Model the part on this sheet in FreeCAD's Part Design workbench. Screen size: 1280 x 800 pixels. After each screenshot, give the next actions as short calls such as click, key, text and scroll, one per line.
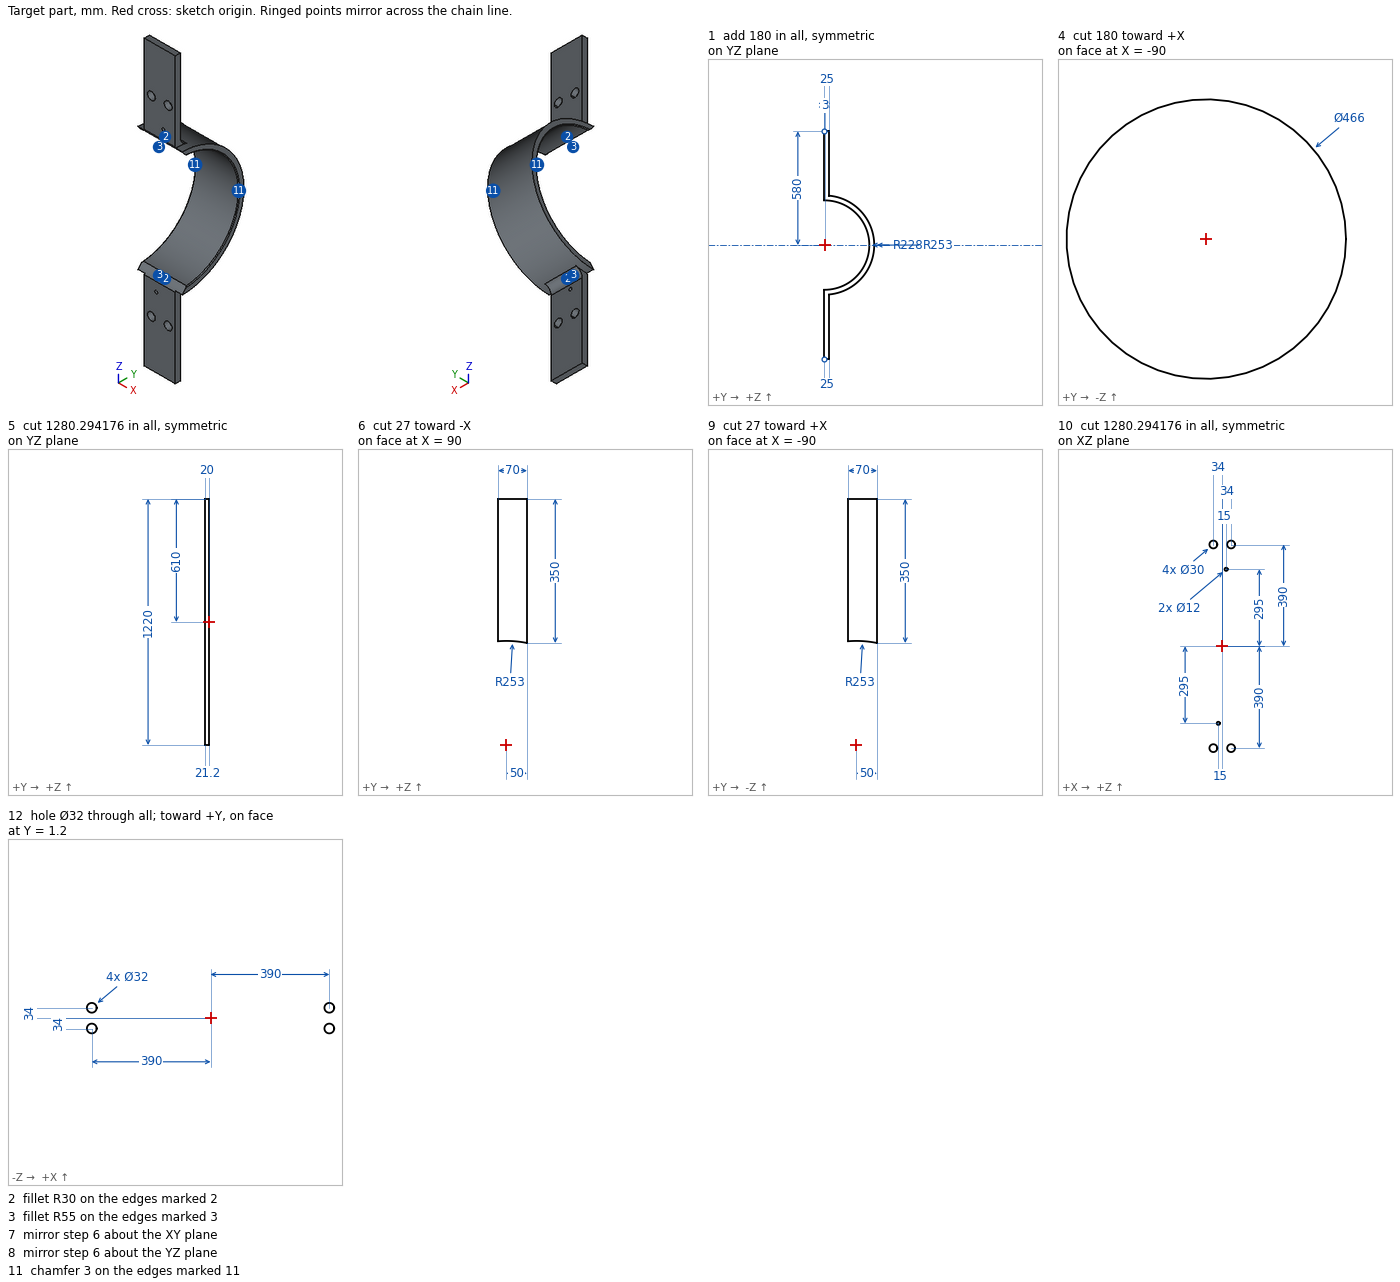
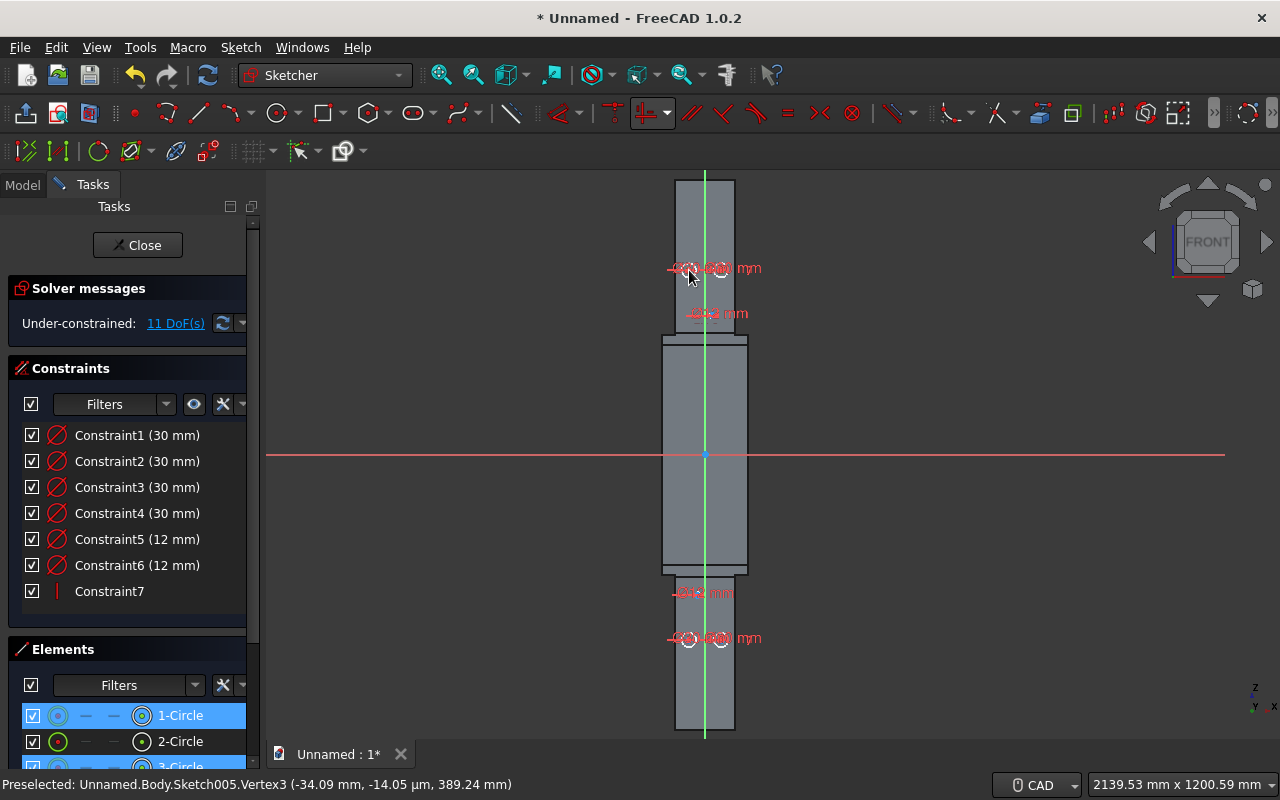
key(h)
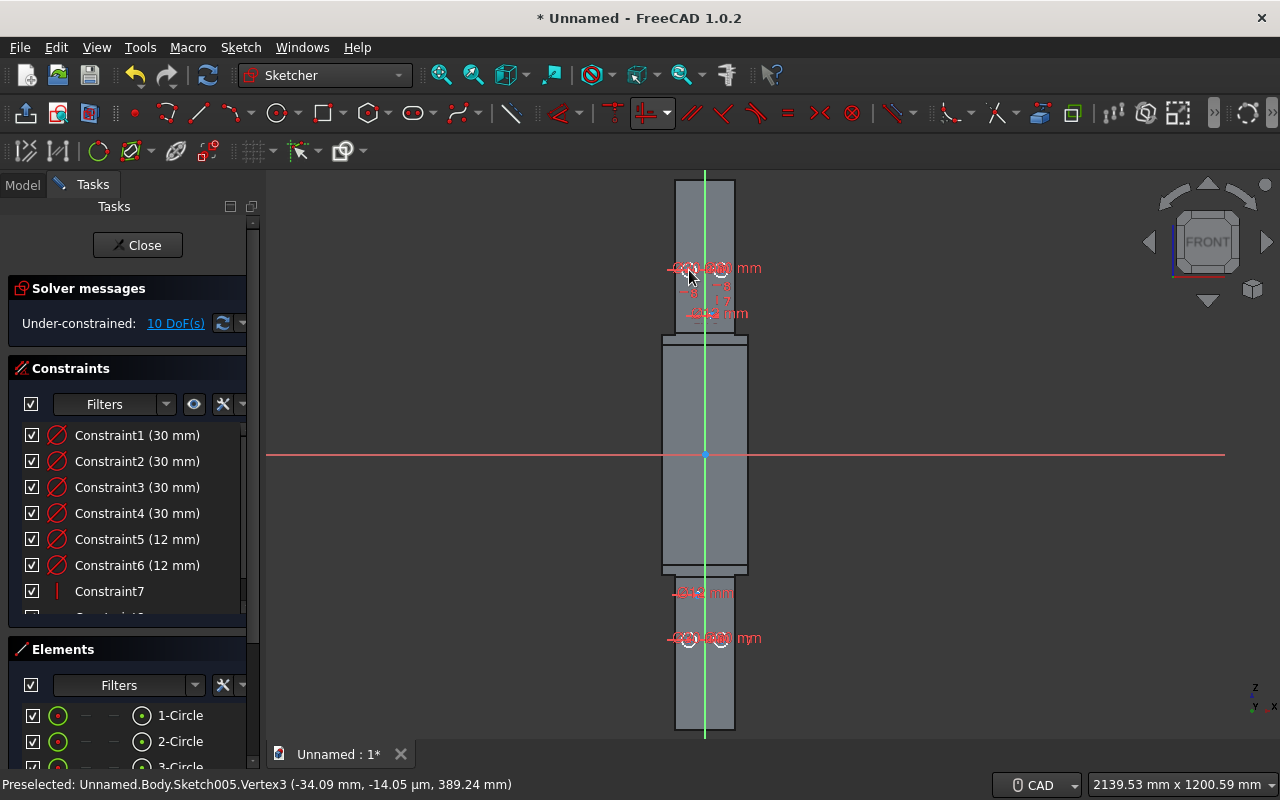
click(689, 270)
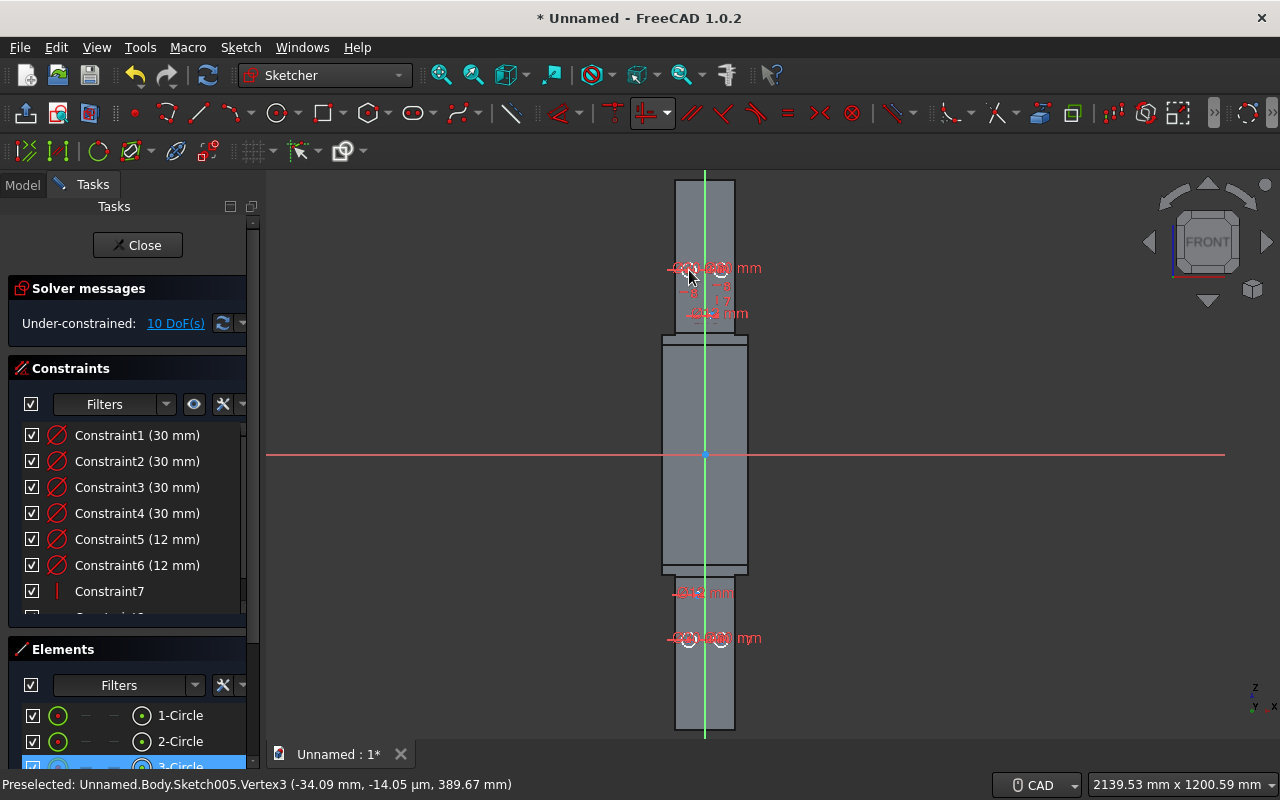
click(689, 640)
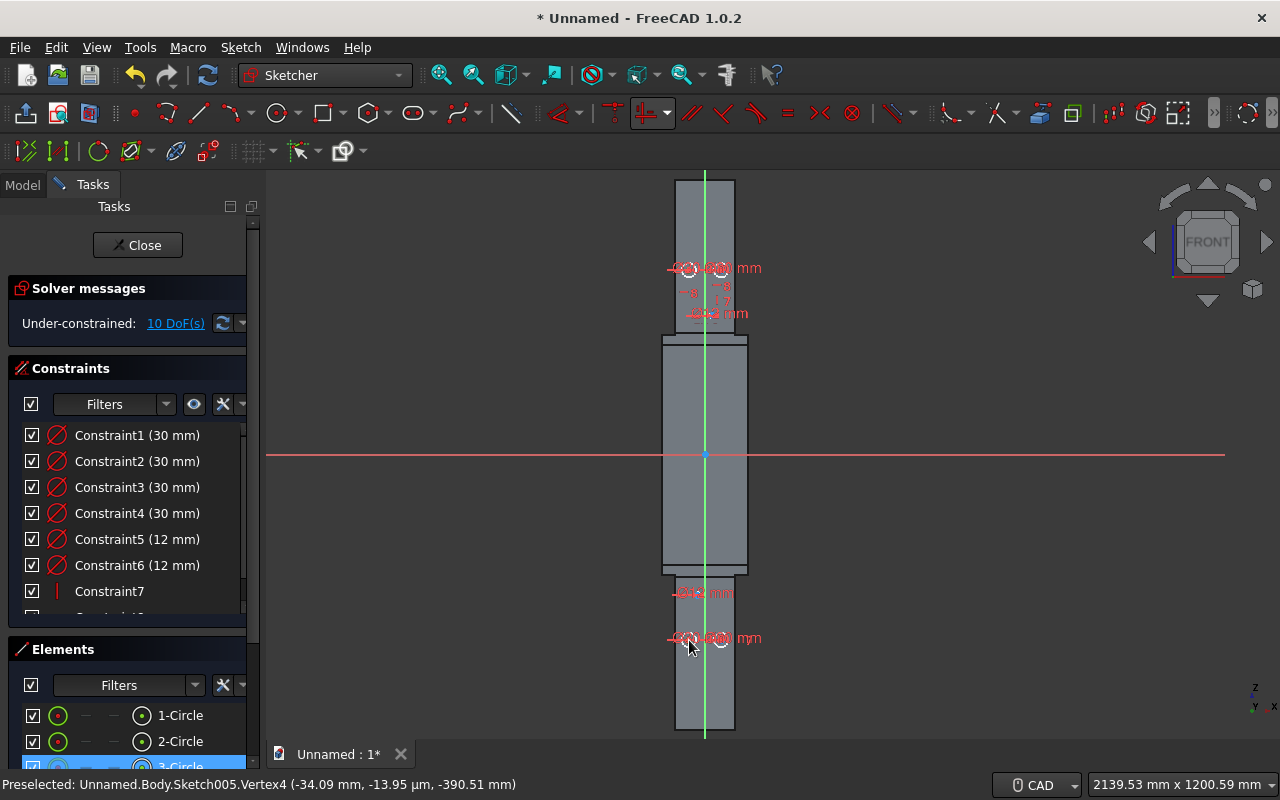
click(670, 114)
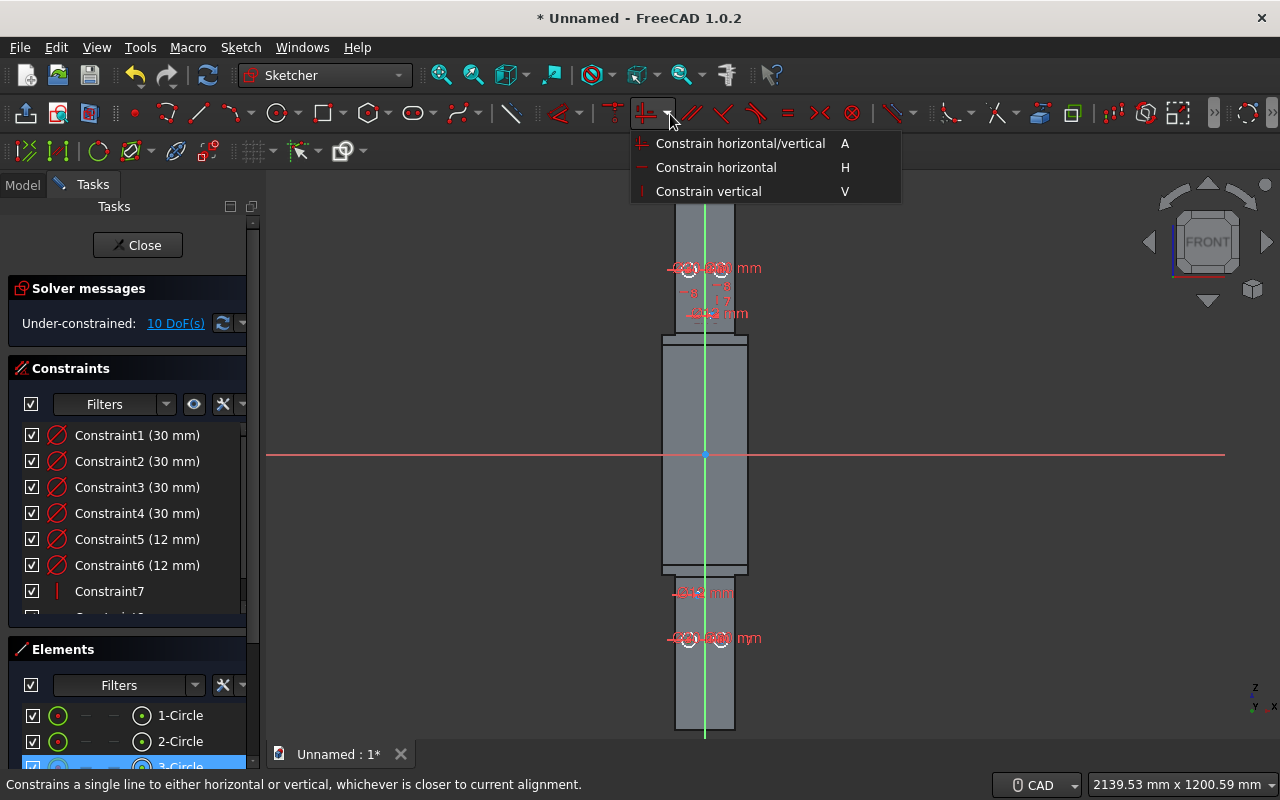
click(766, 191)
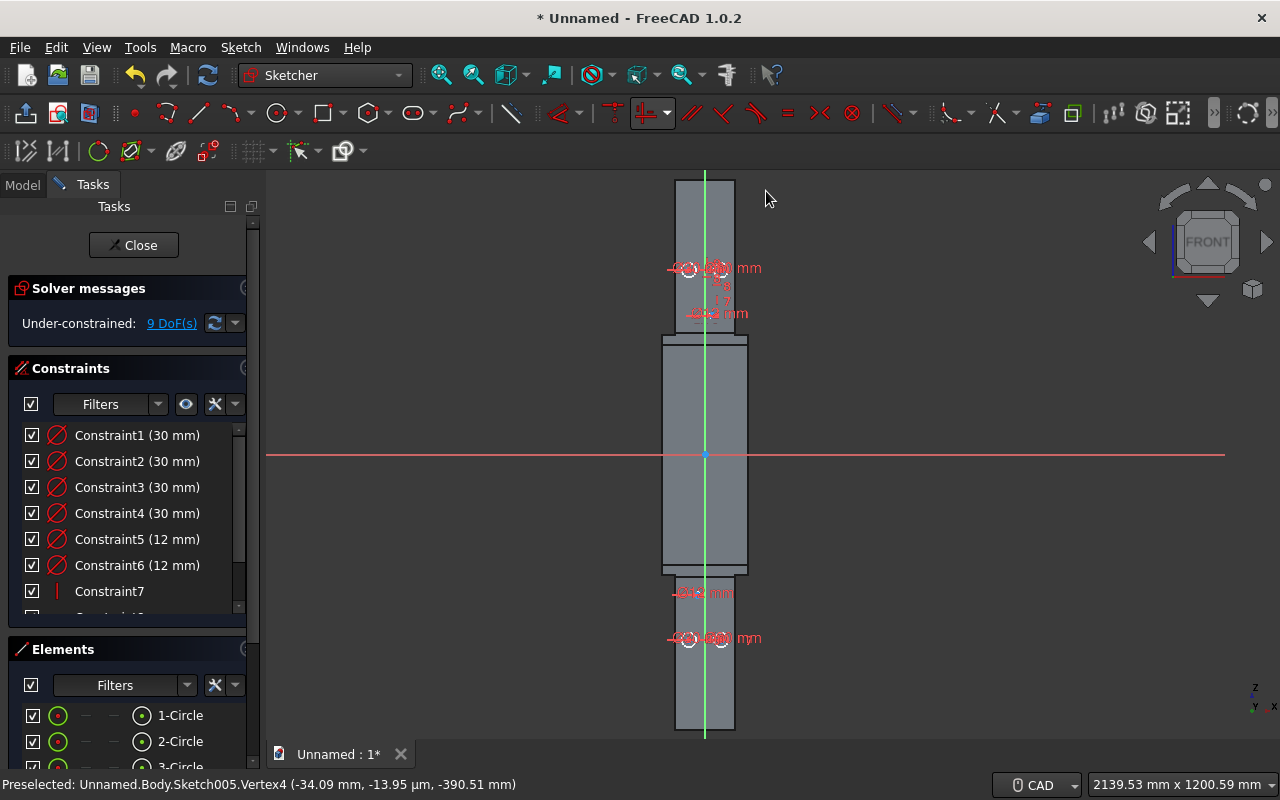
click(723, 642)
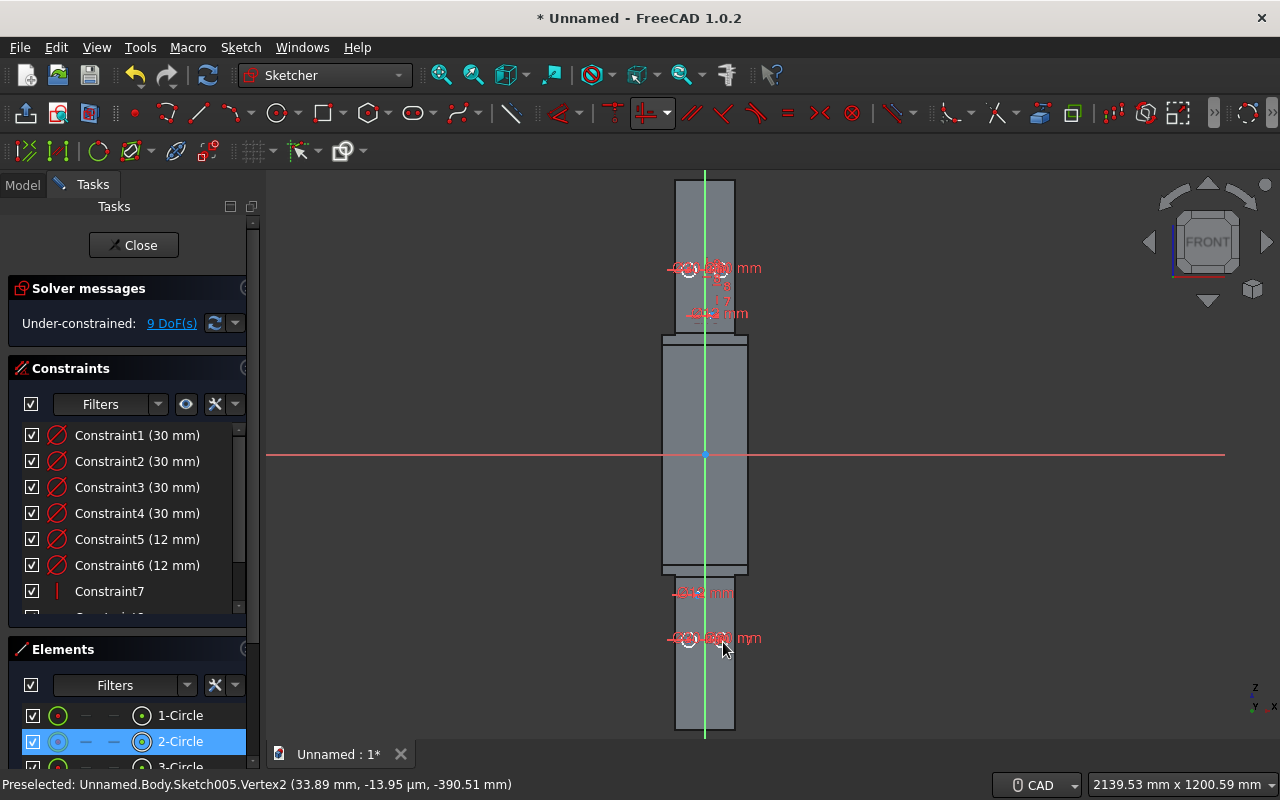
click(689, 640)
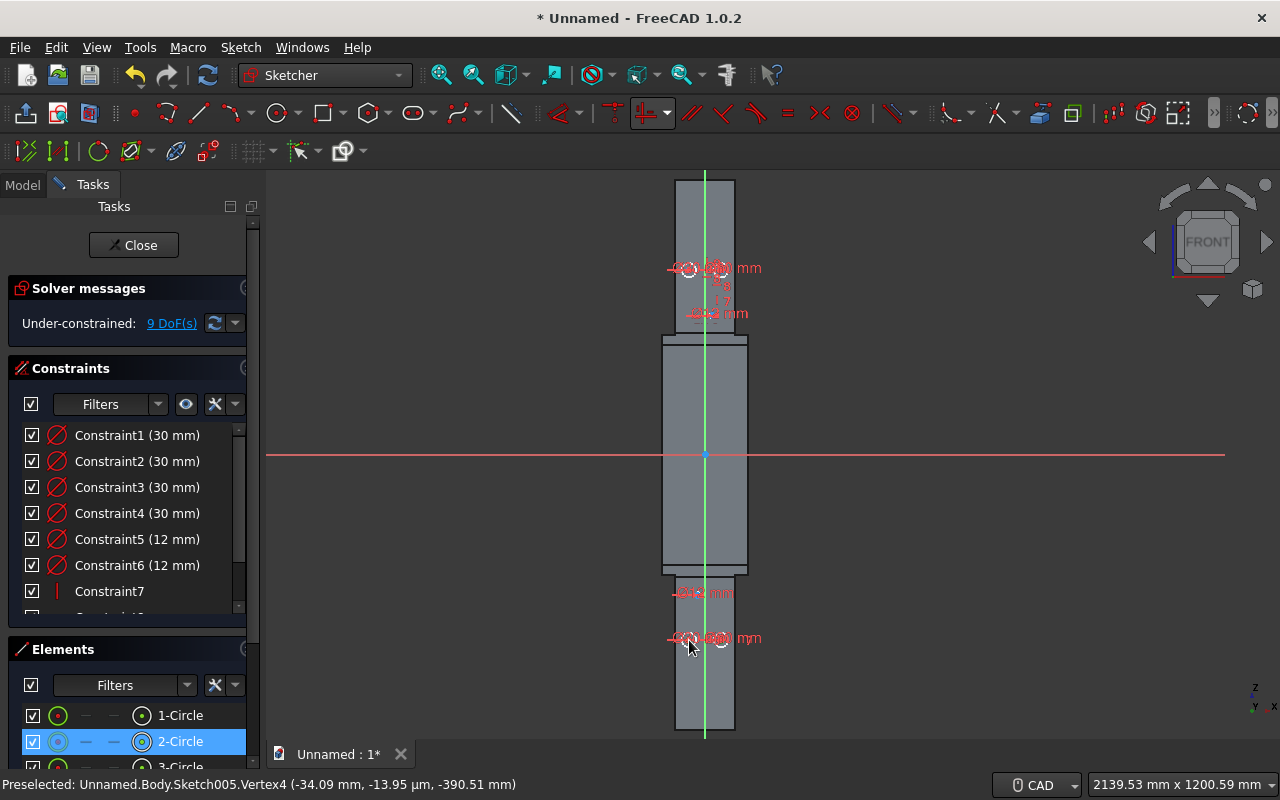
click(670, 114)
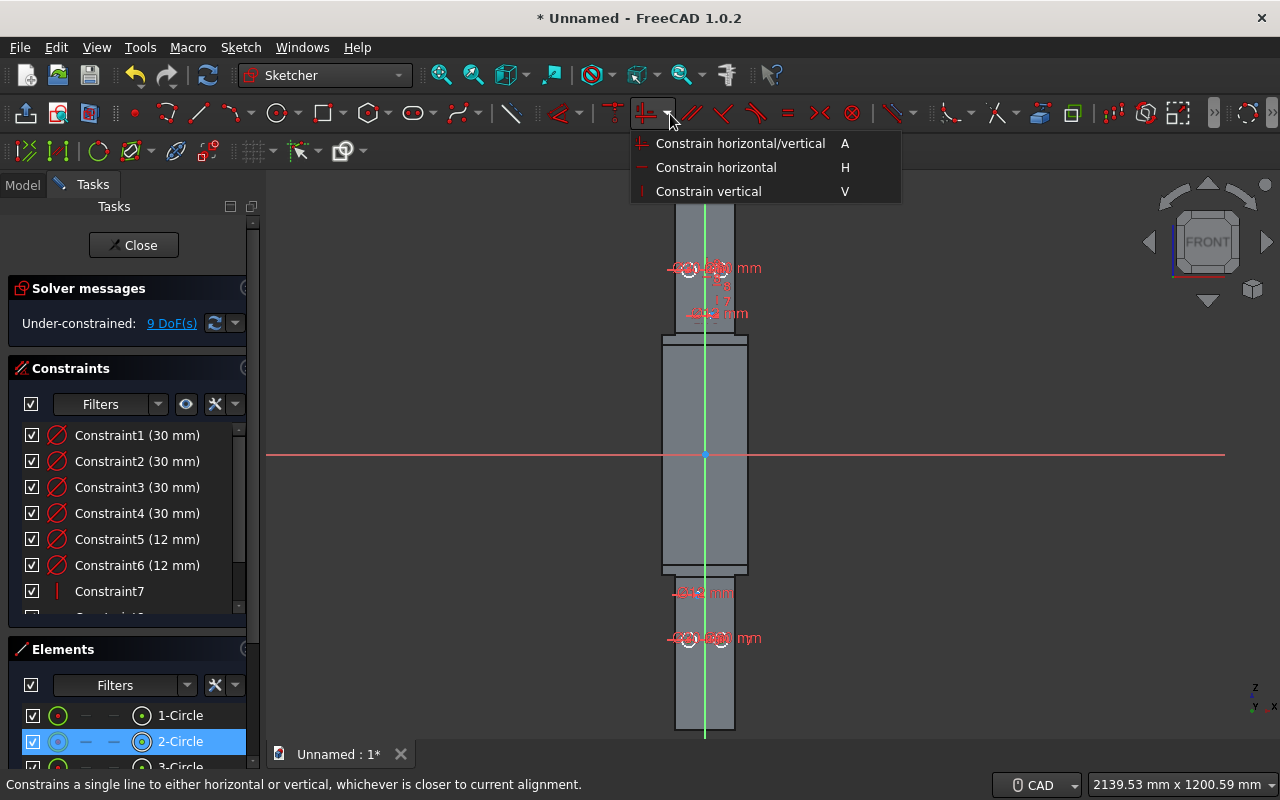
click(766, 167)